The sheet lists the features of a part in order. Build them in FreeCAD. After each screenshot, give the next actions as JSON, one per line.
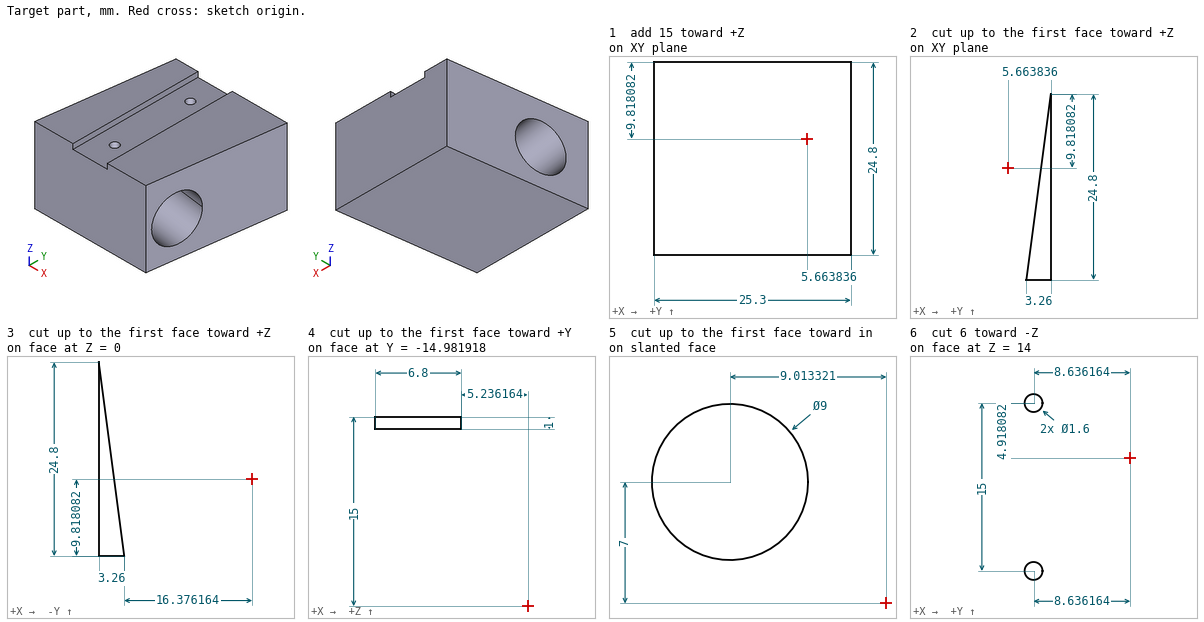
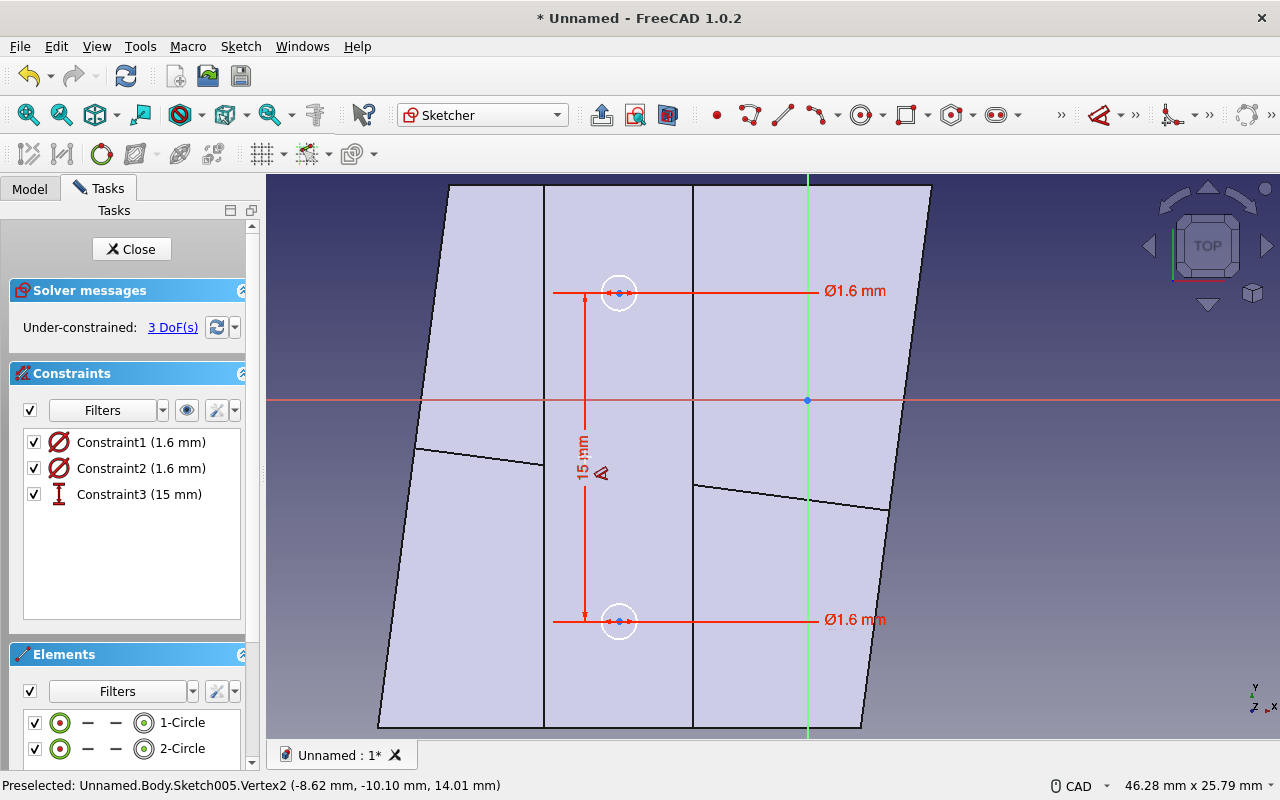
{"action": "left_click", "coordinate": [619, 293]}
{"action": "left_click", "coordinate": [714, 259]}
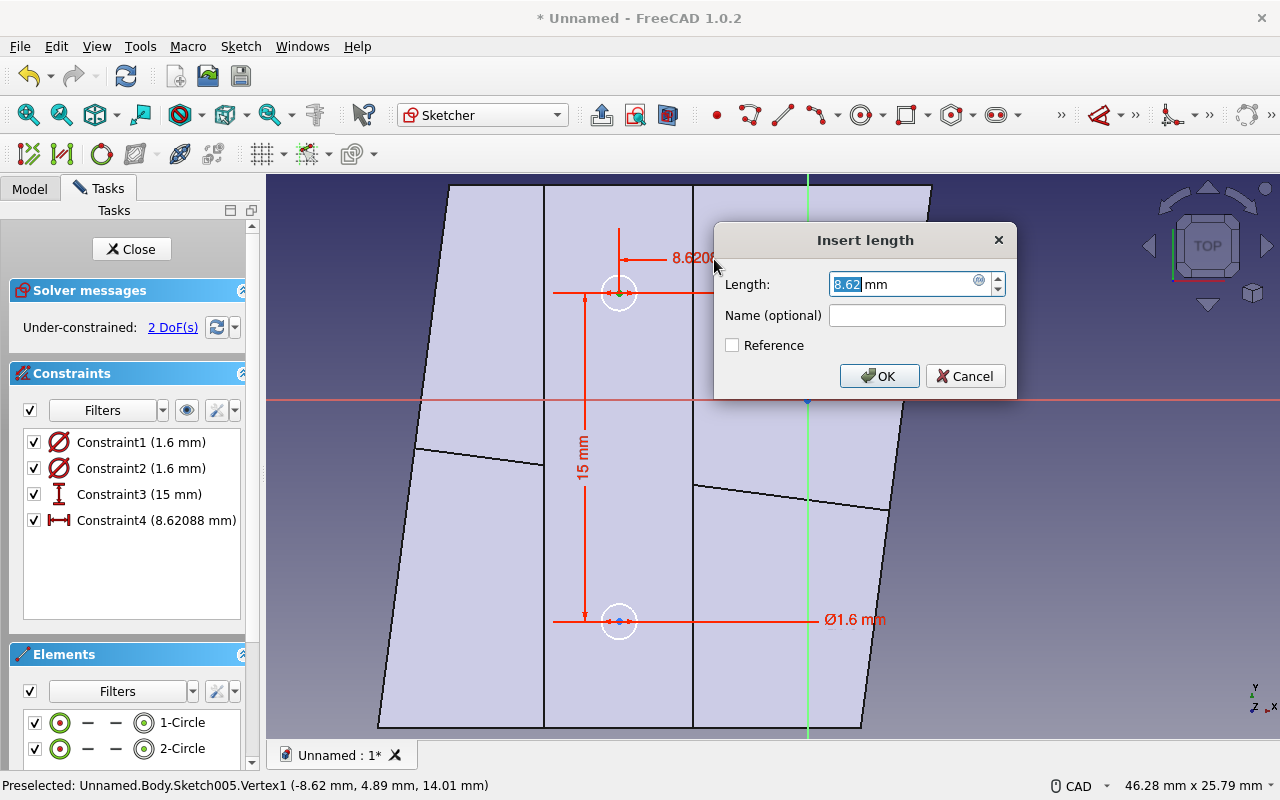
{"action": "type", "text": "8.636164"}
{"action": "key", "text": "Return"}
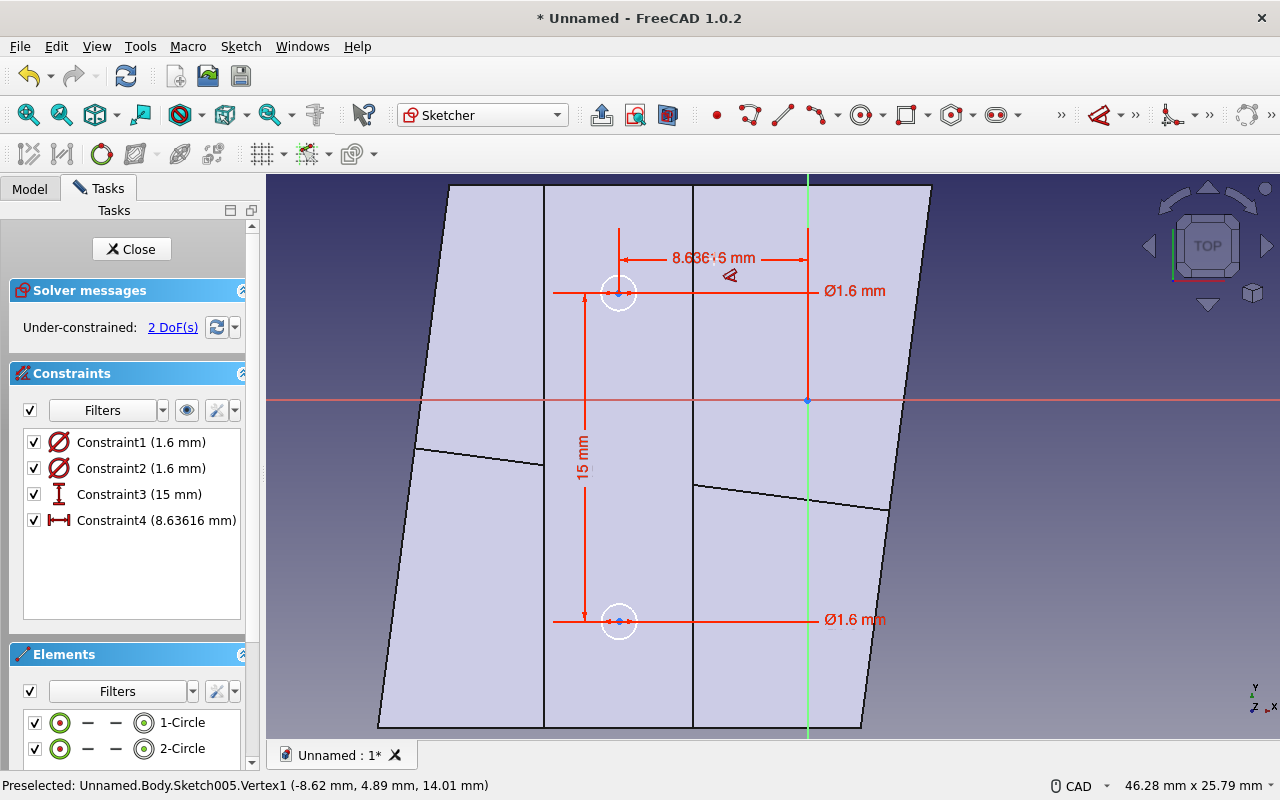
{"action": "left_click", "coordinate": [619, 293]}
{"action": "left_click", "coordinate": [842, 347]}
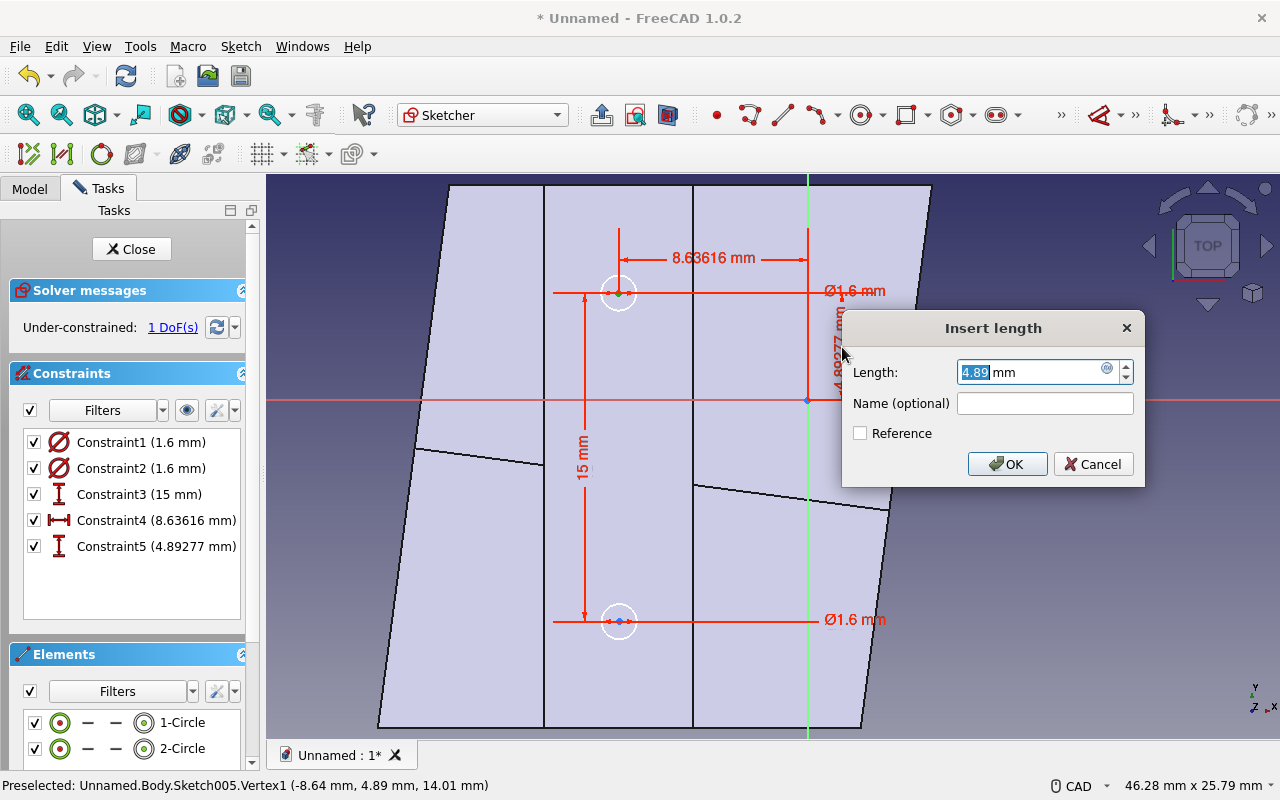
{"action": "type", "text": "4.918082"}
{"action": "key", "text": "Return"}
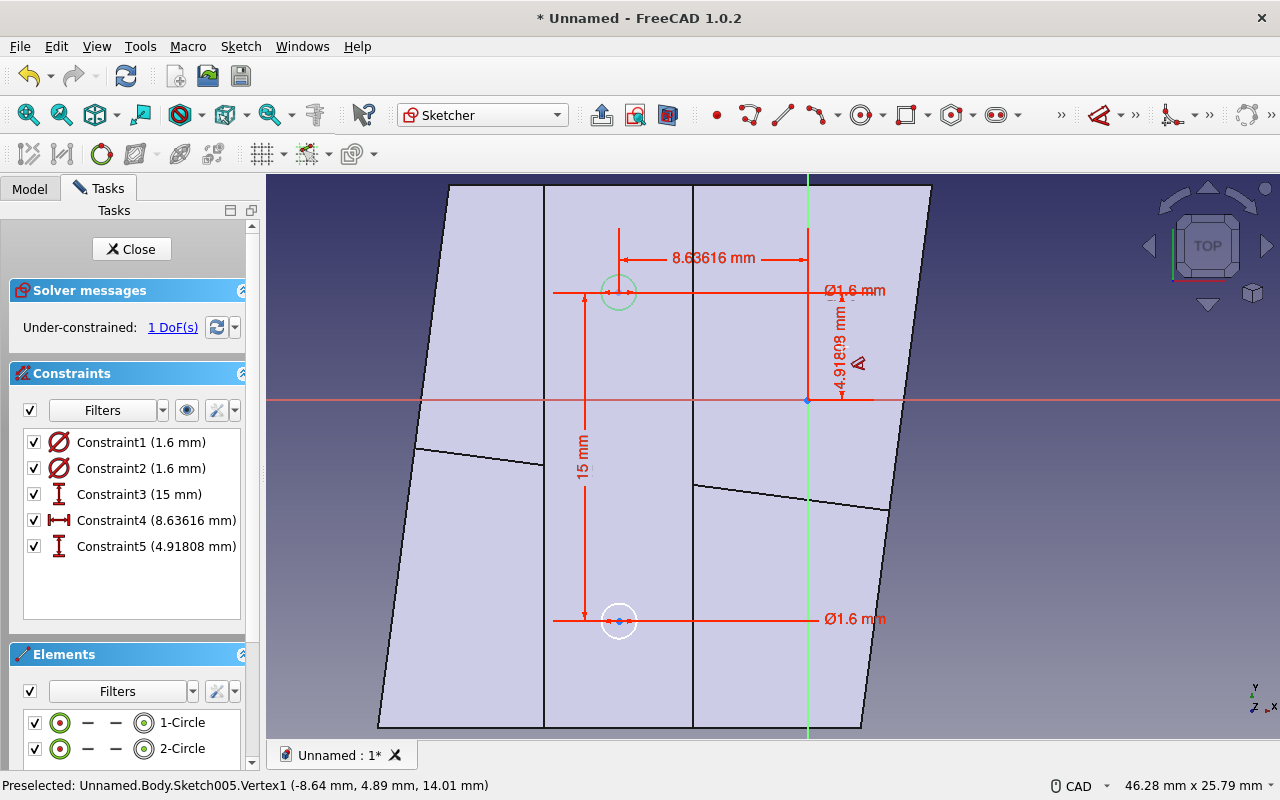
{"action": "left_click", "coordinate": [619, 621]}
{"action": "left_click", "coordinate": [714, 655]}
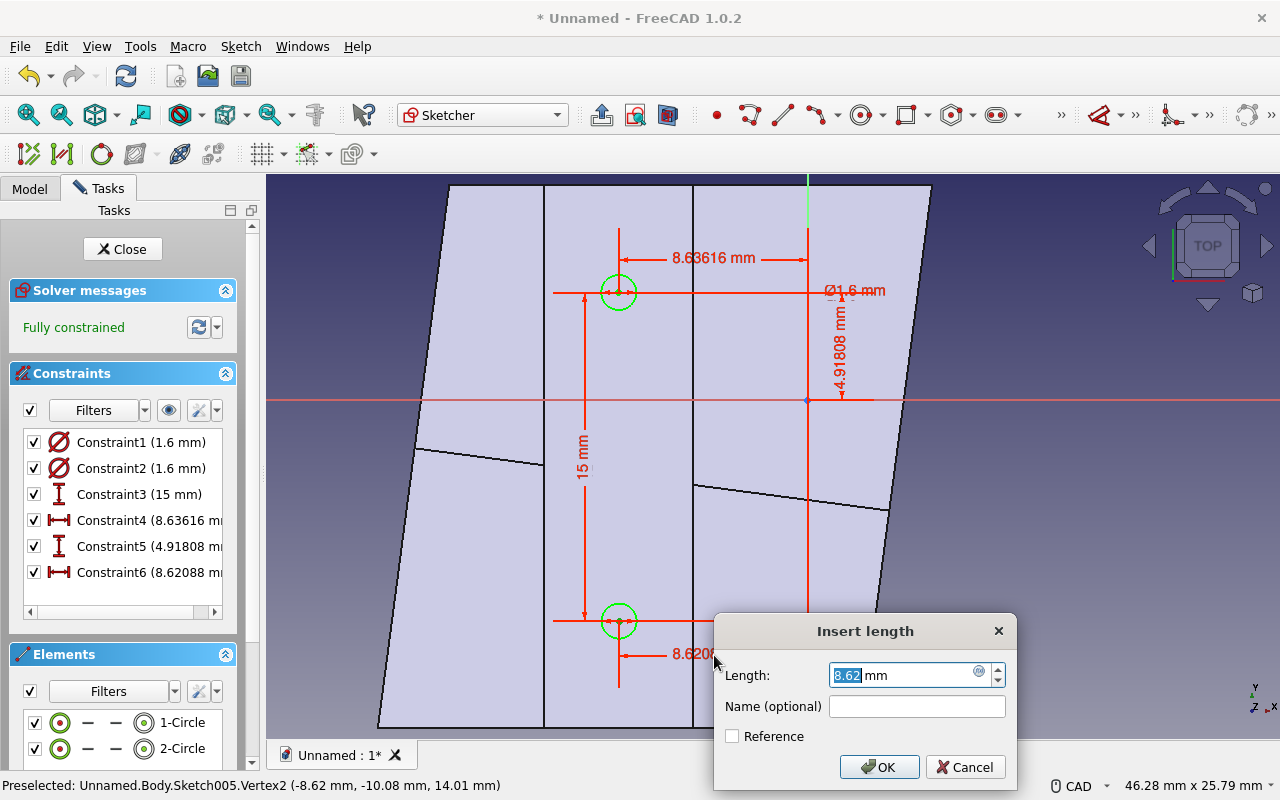
{"action": "type", "text": "8.636164"}
{"action": "key", "text": "Return"}
{"action": "key", "text": "Escape"}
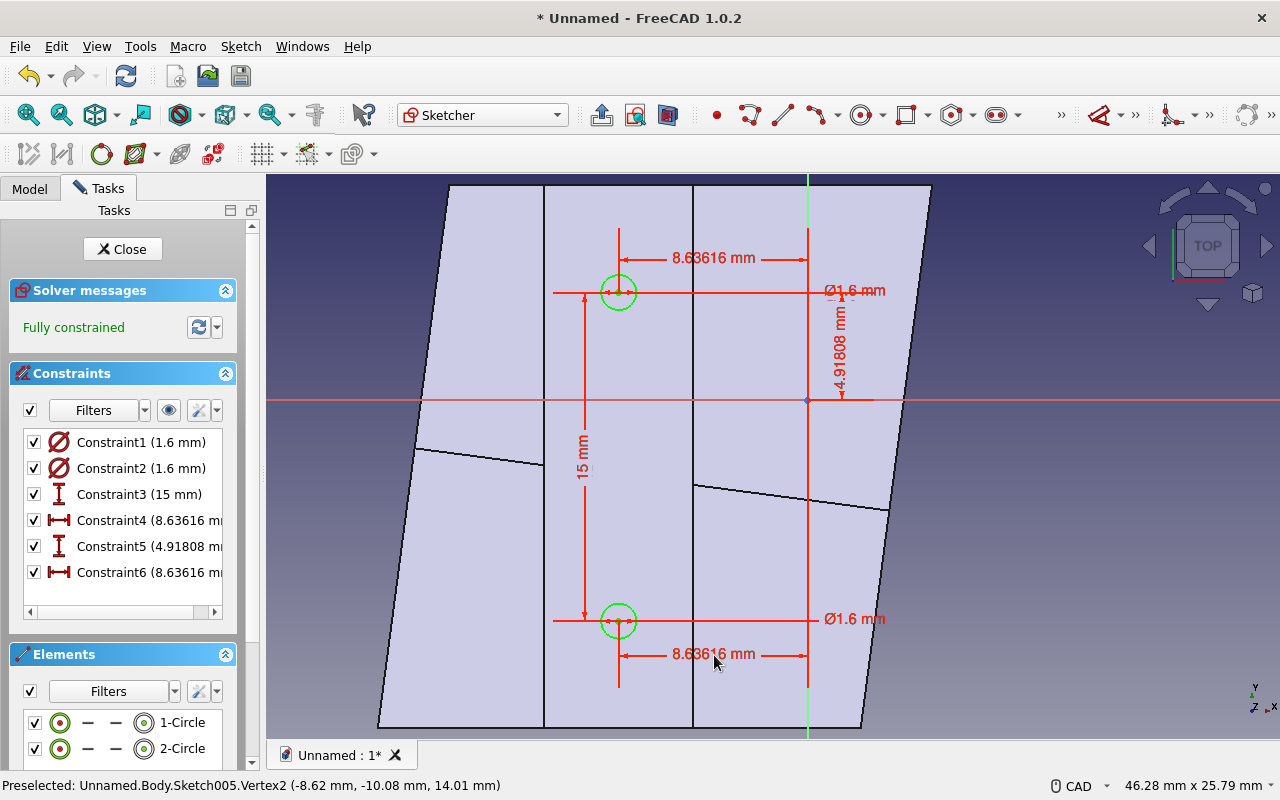
{"action": "left_click", "coordinate": [123, 249]}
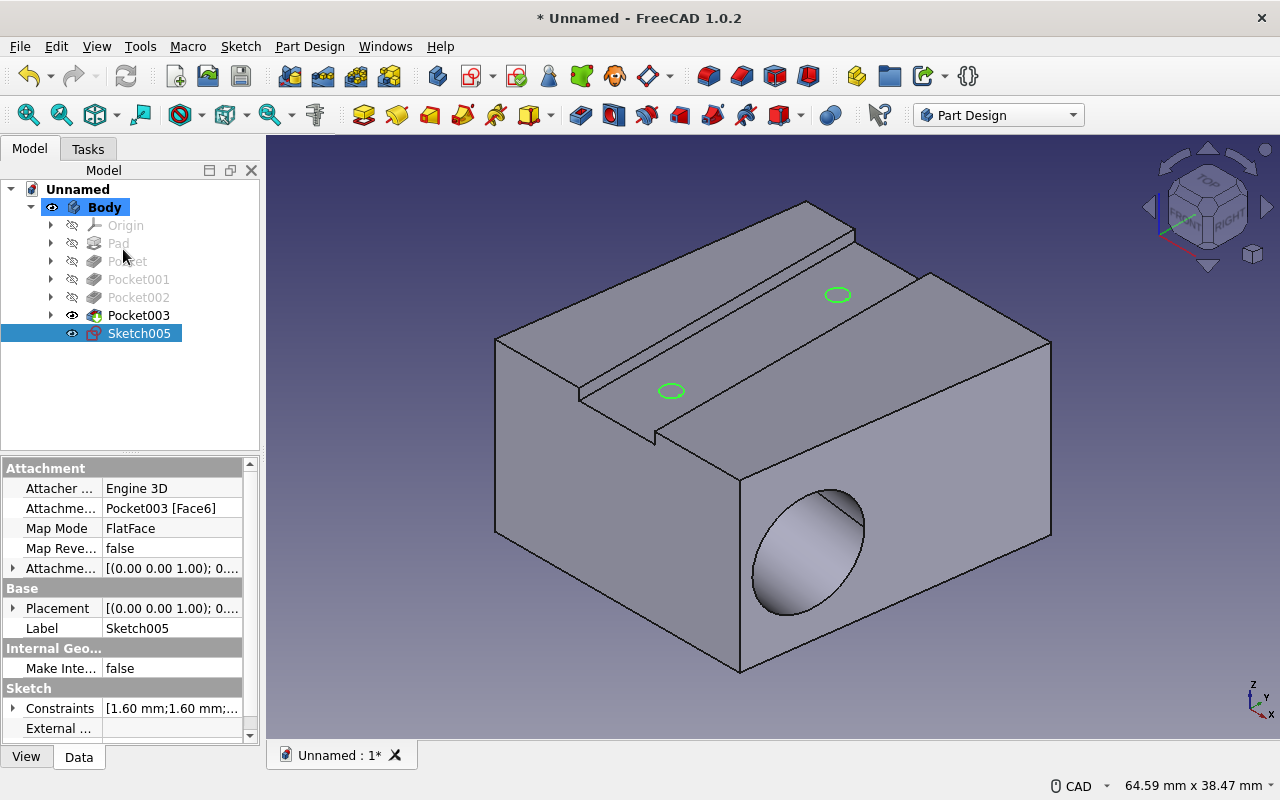
{"action": "left_click", "coordinate": [581, 116]}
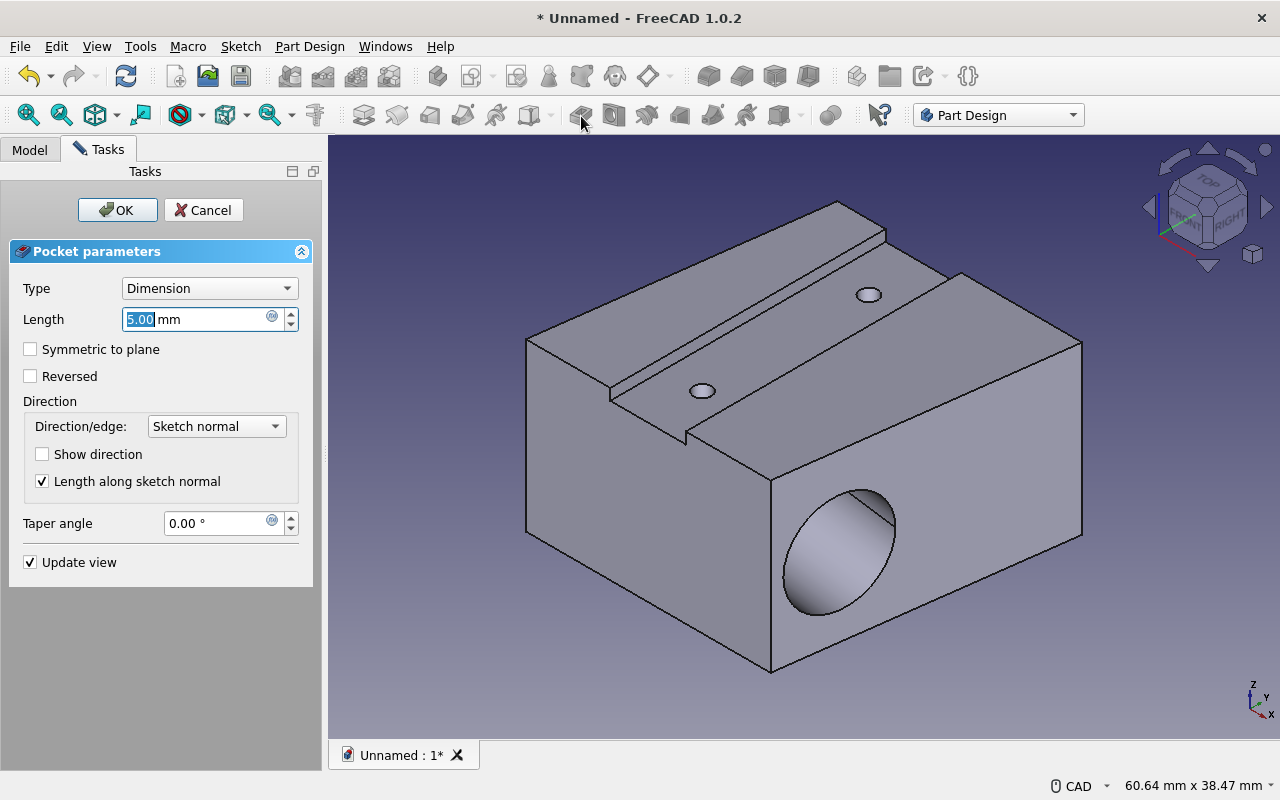
{"action": "type", "text": "6"}
{"action": "key", "text": "Tab"}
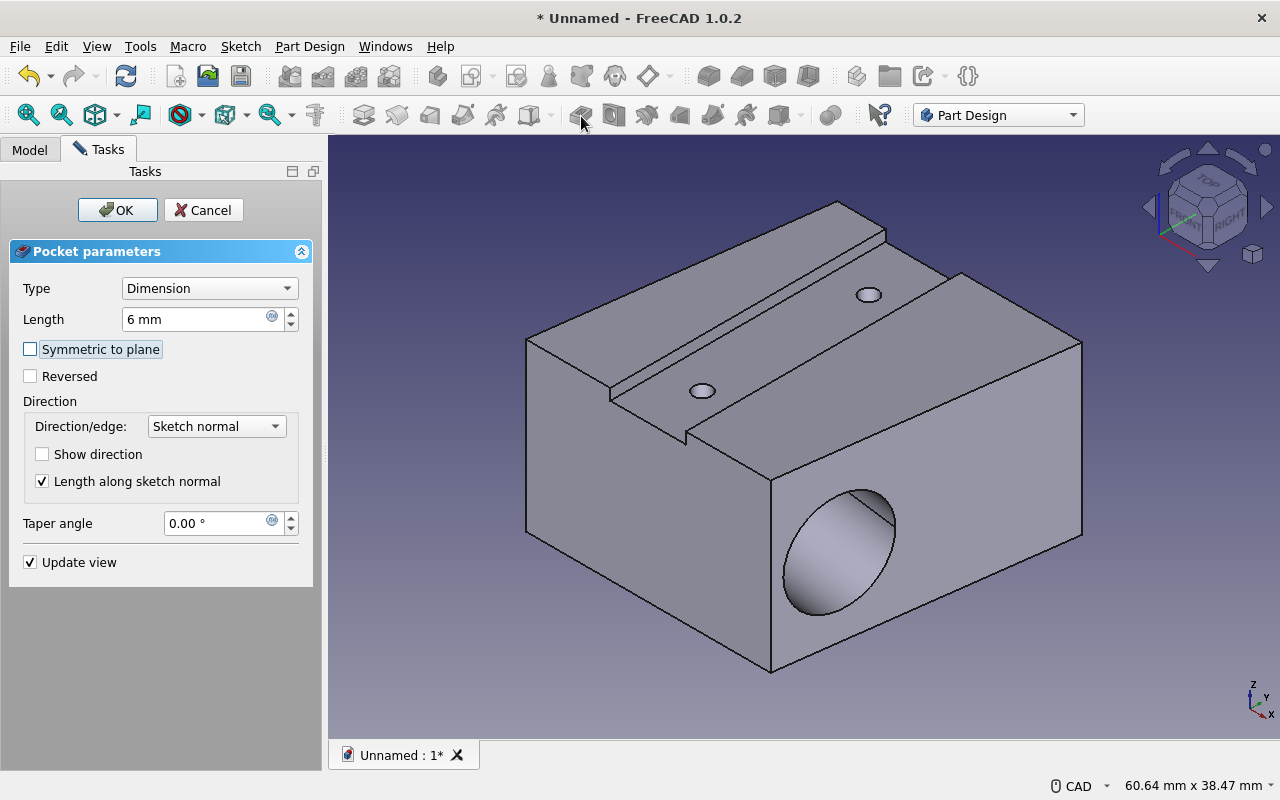
{"action": "left_click", "coordinate": [118, 210]}